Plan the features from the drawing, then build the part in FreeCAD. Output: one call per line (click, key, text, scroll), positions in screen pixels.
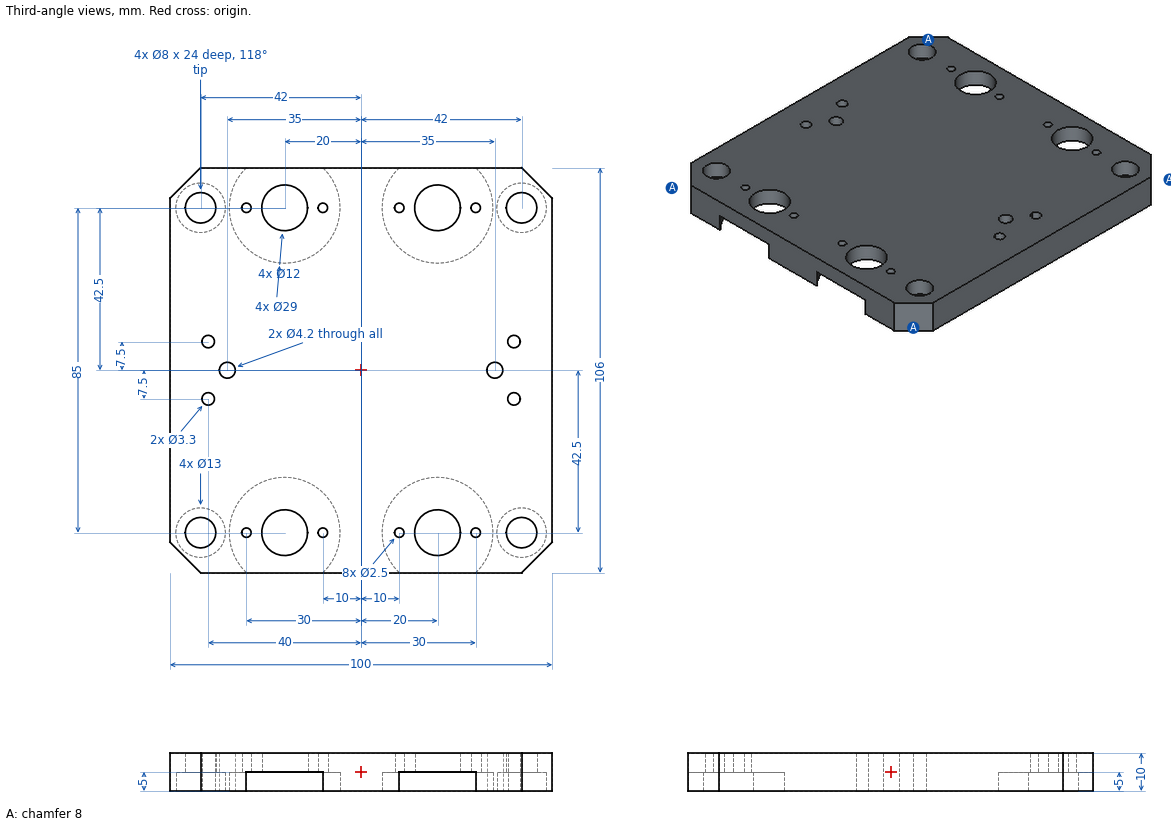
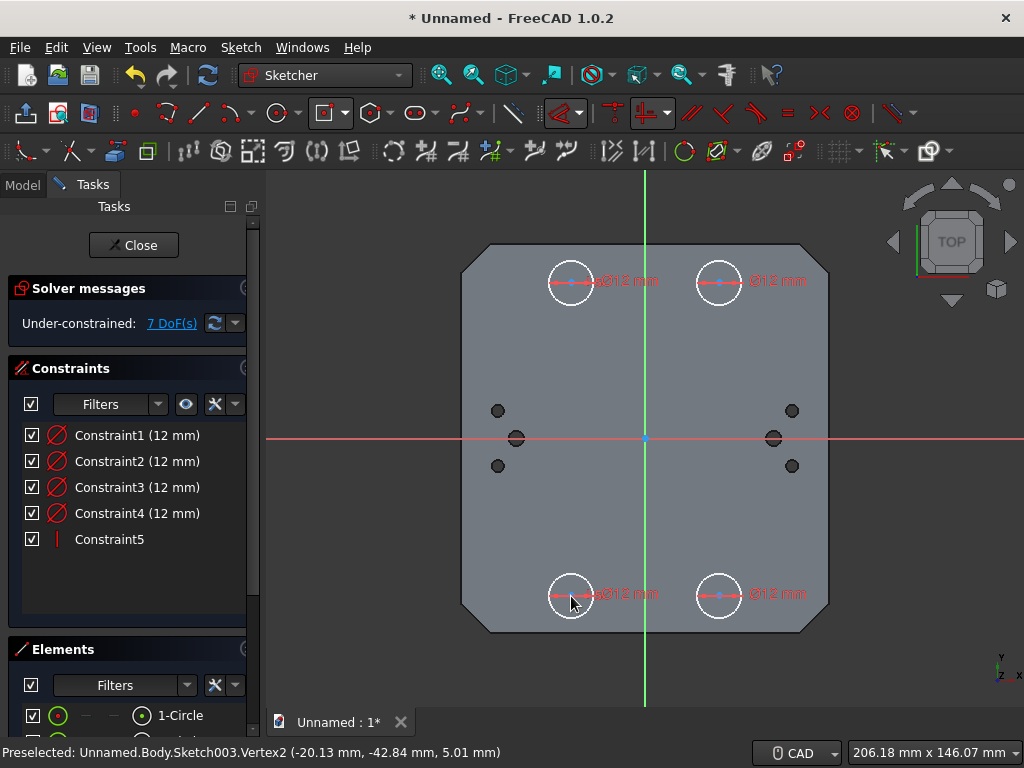
click(571, 596)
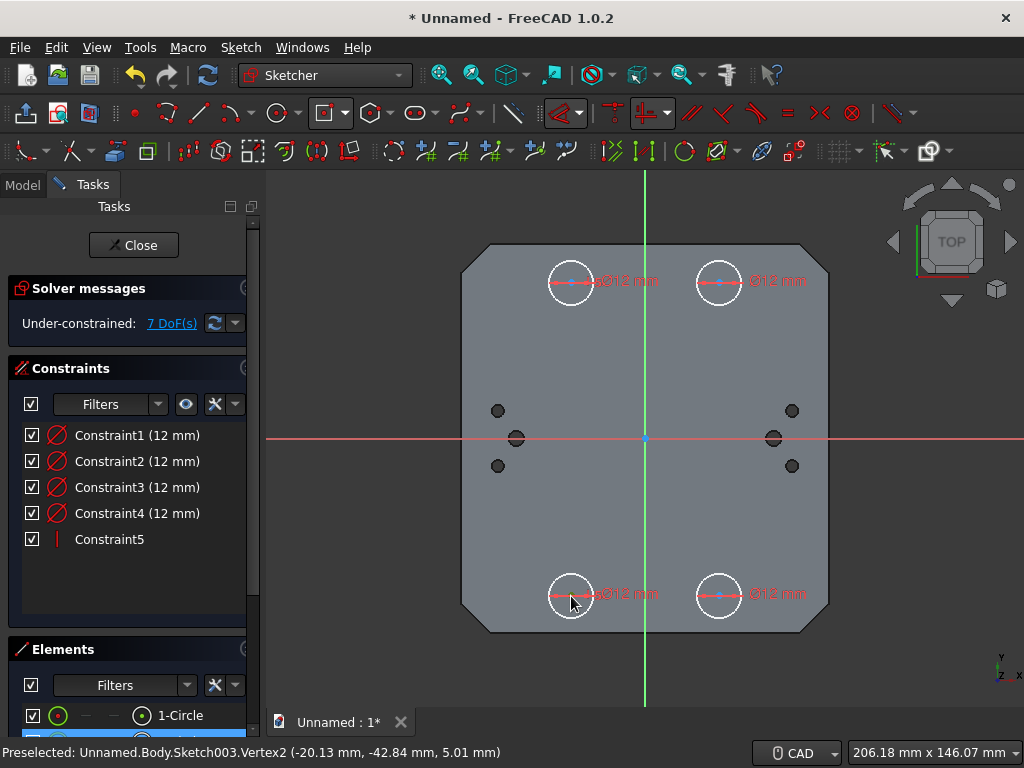
click(719, 596)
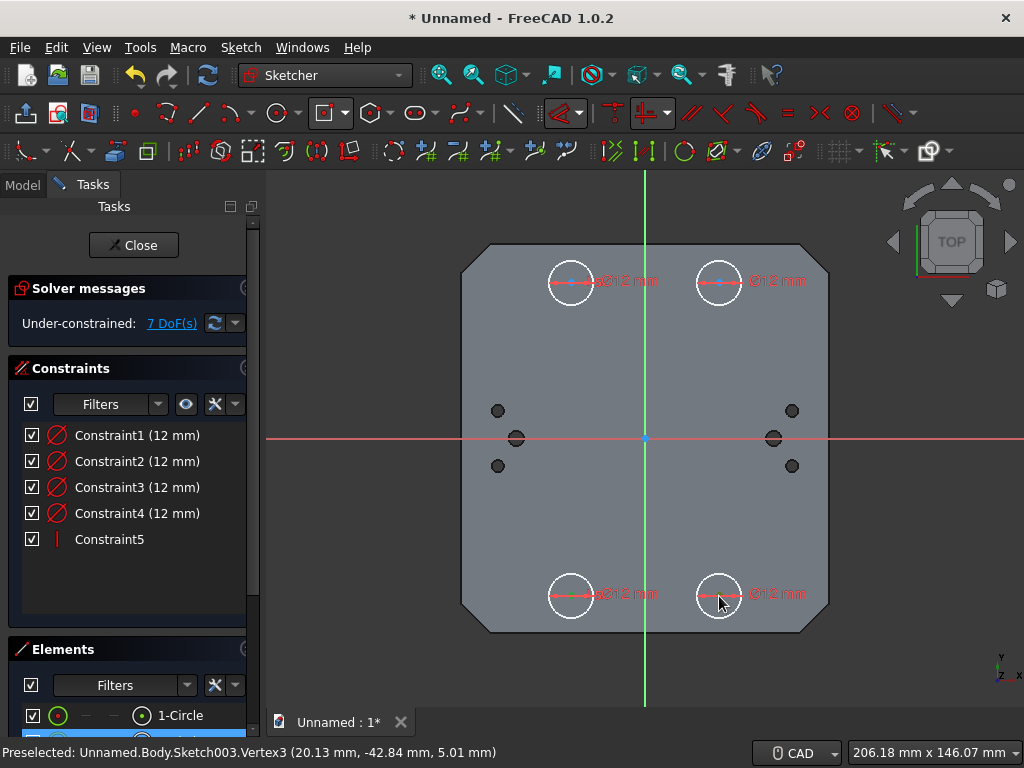
click(670, 114)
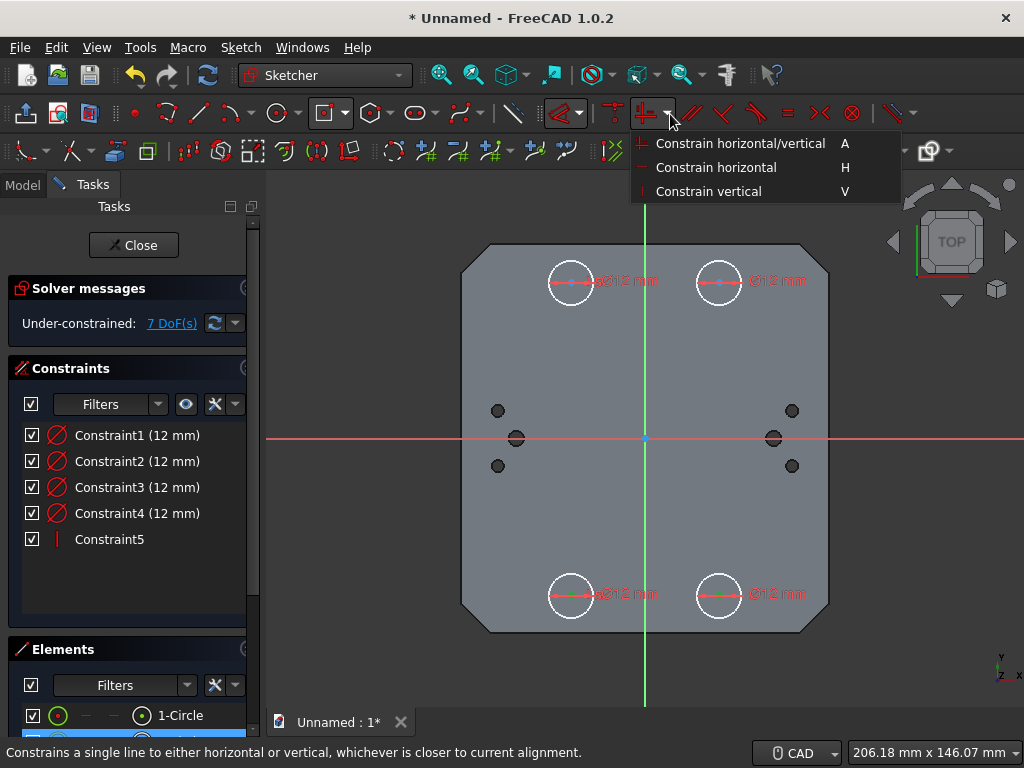
click(766, 167)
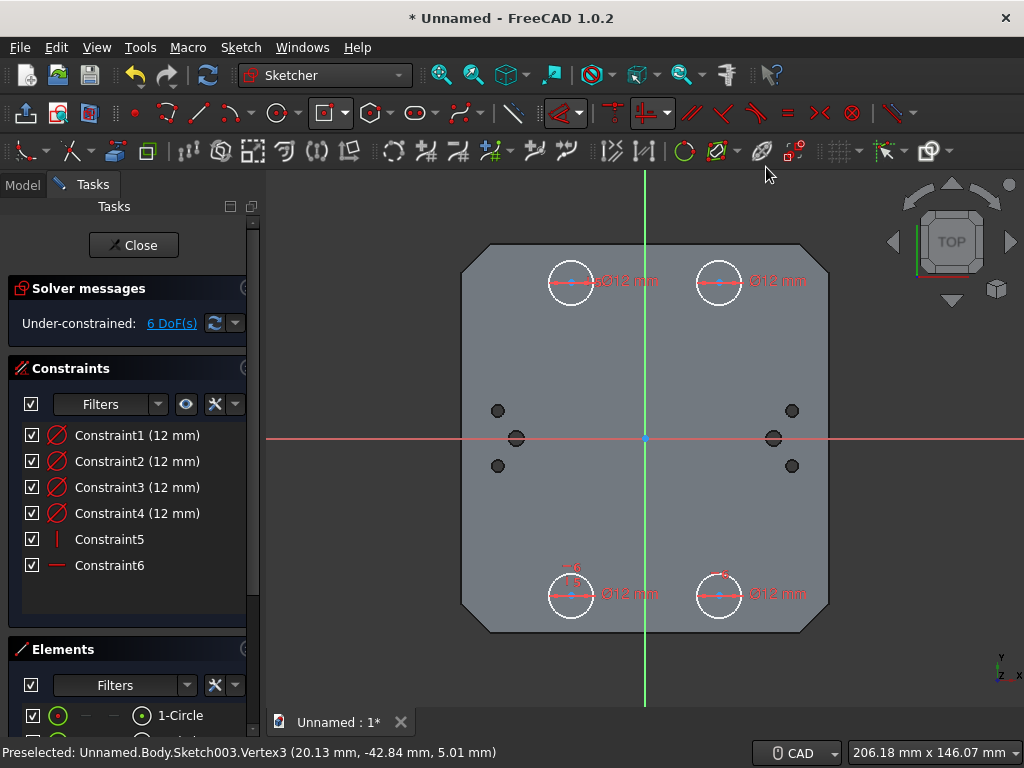
click(719, 596)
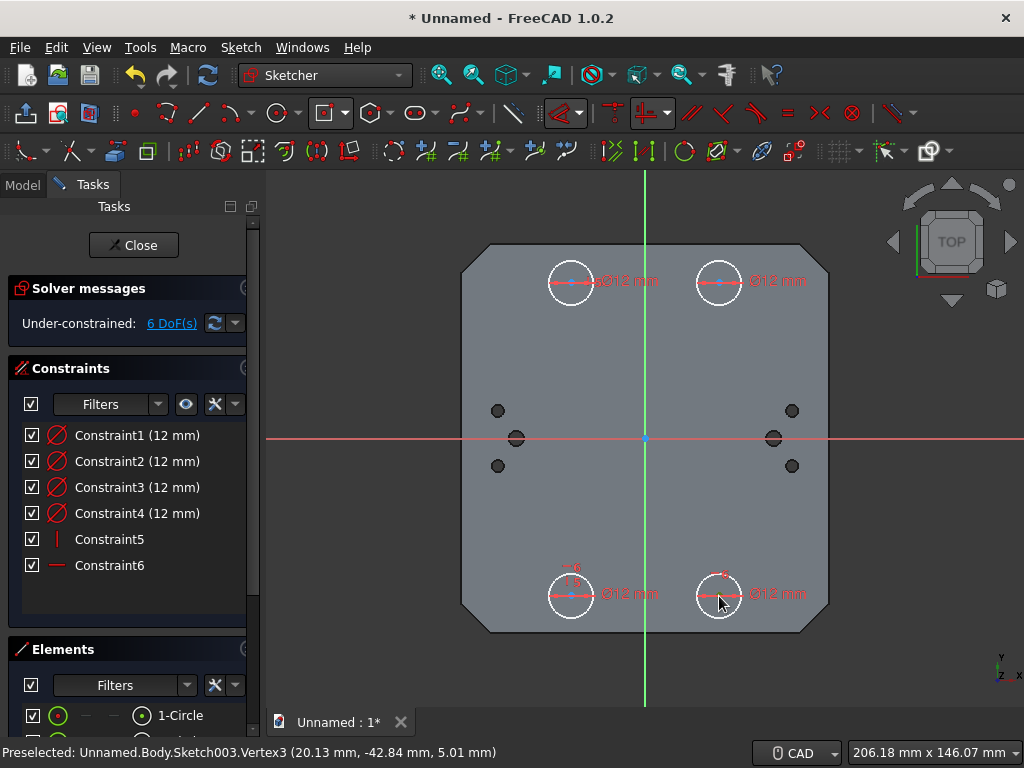
click(719, 283)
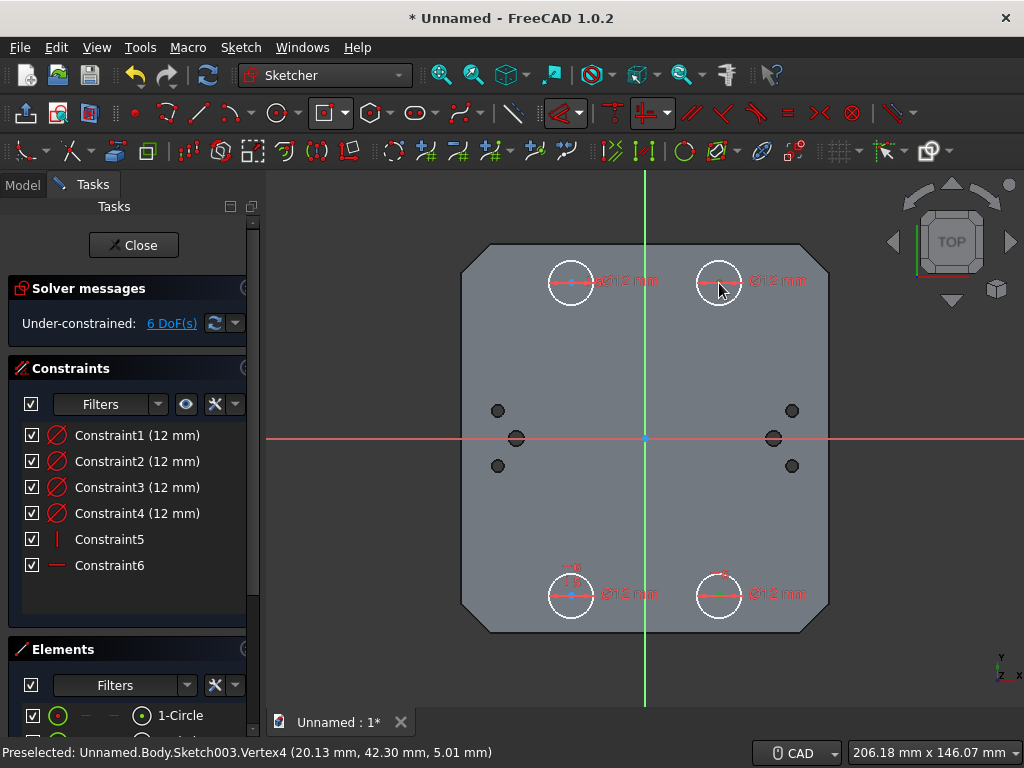
key(v)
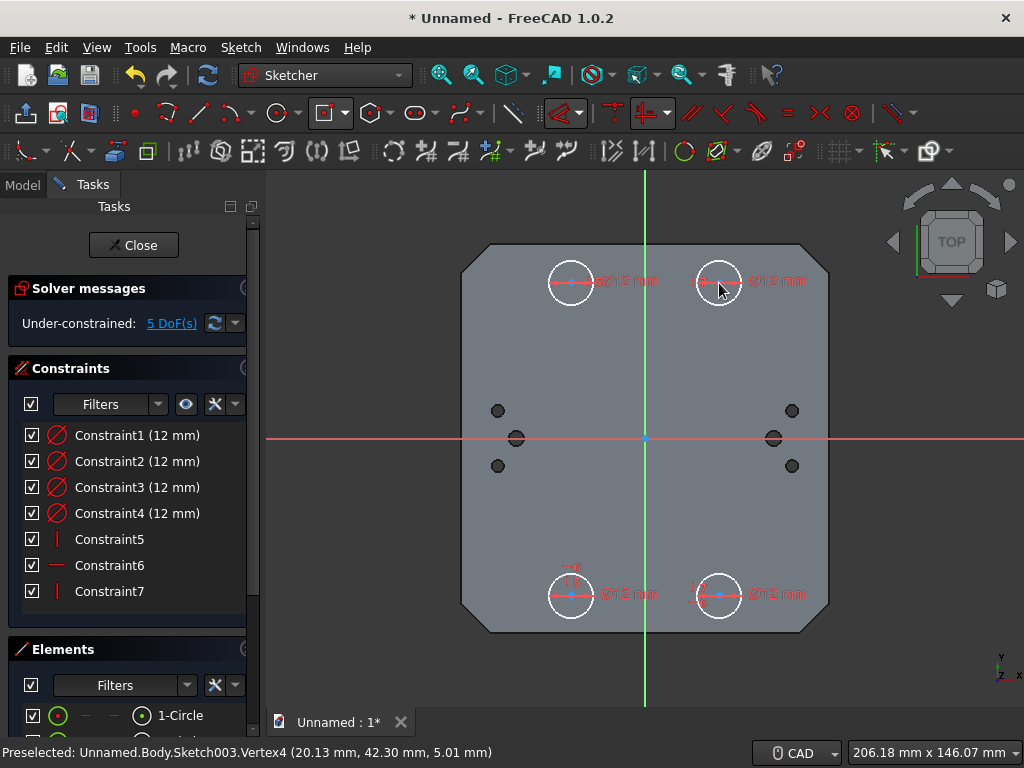
click(571, 283)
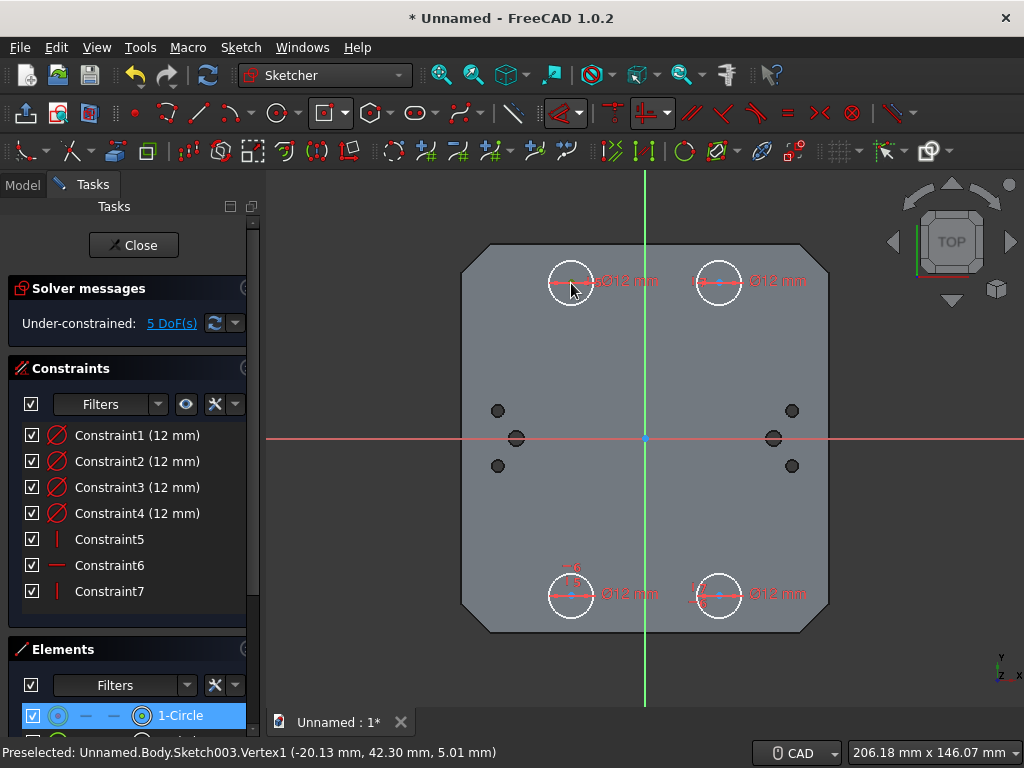
click(719, 283)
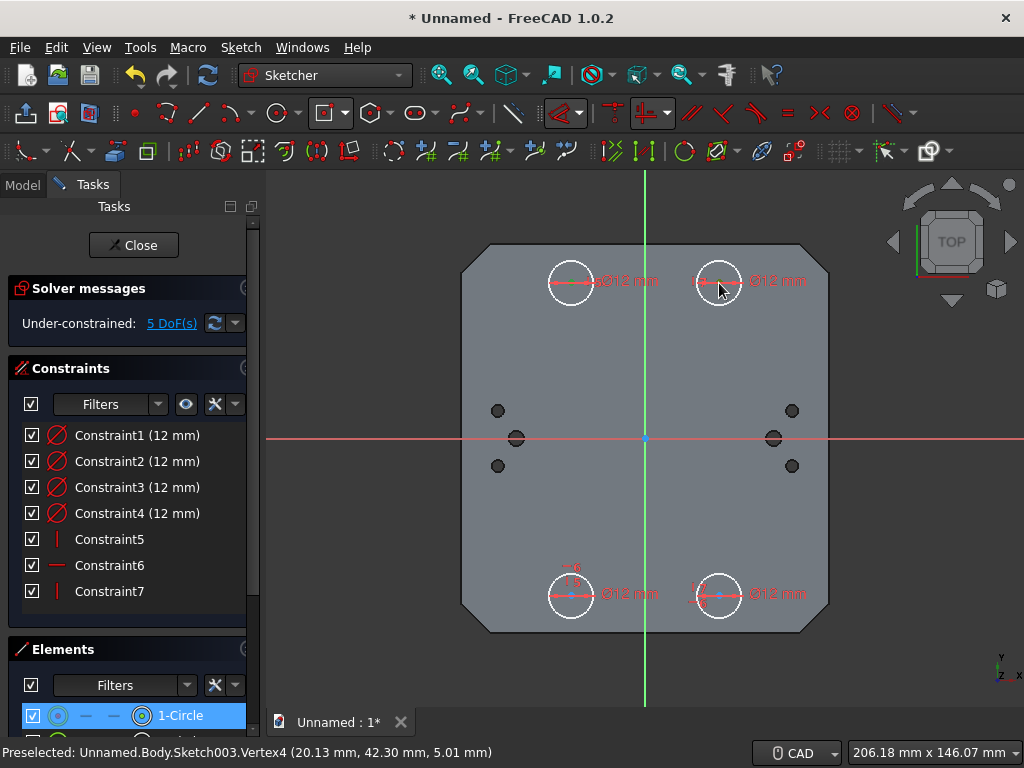
click(670, 114)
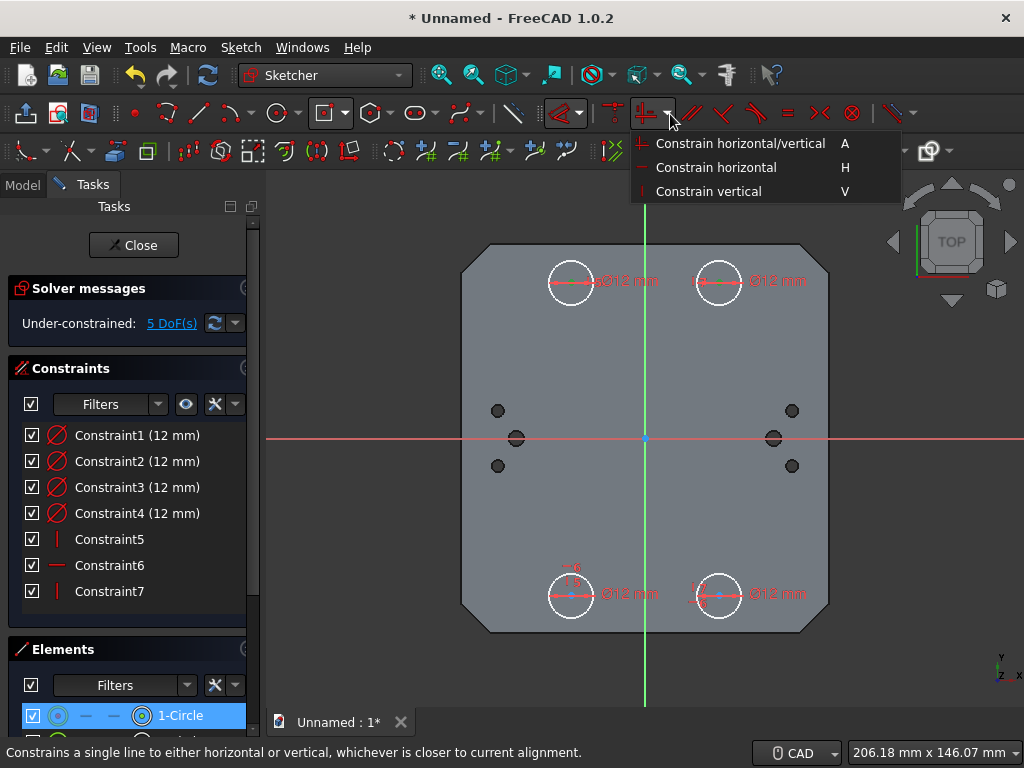
click(766, 167)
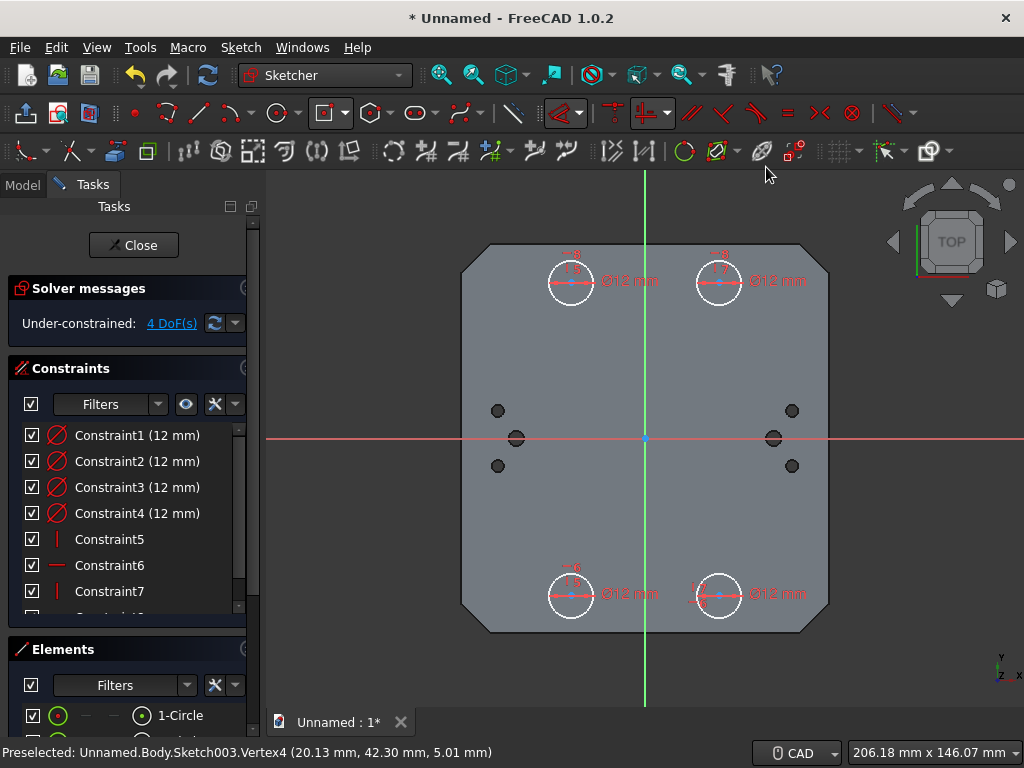
click(571, 283)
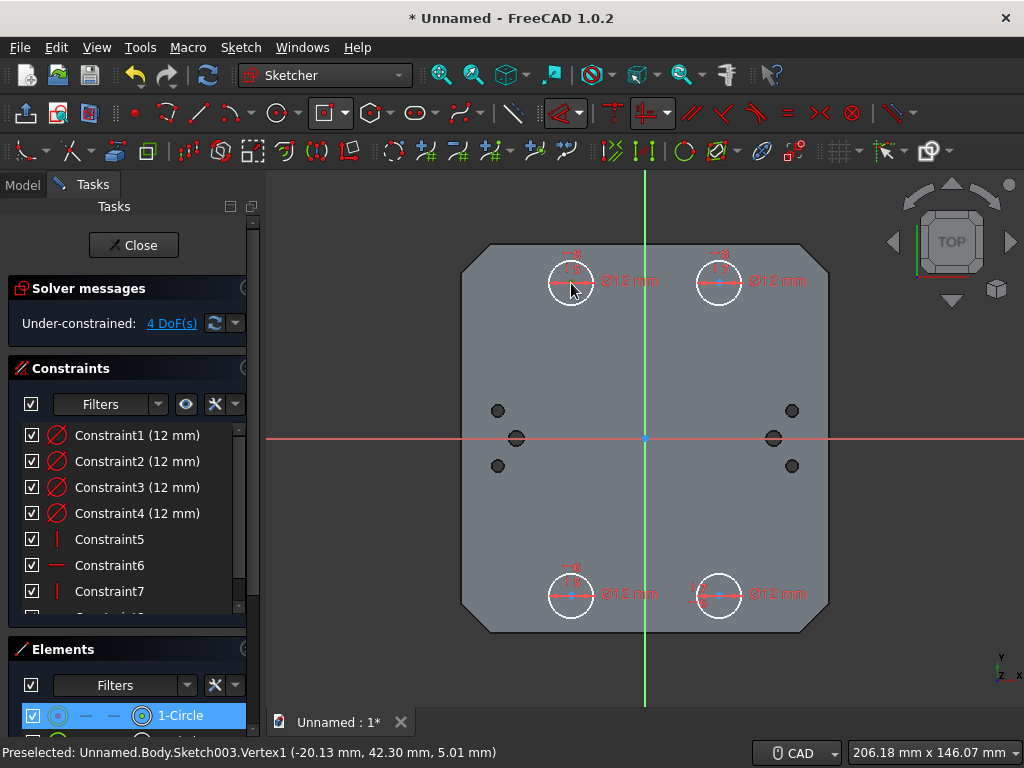
key(l)